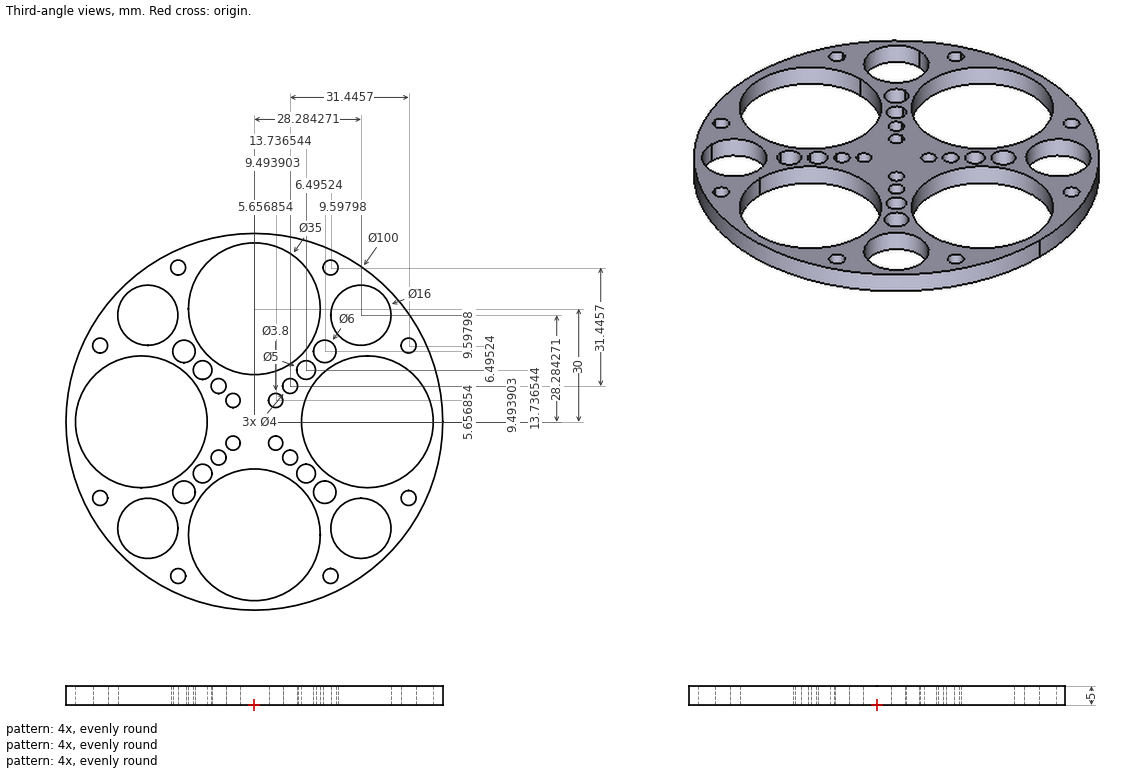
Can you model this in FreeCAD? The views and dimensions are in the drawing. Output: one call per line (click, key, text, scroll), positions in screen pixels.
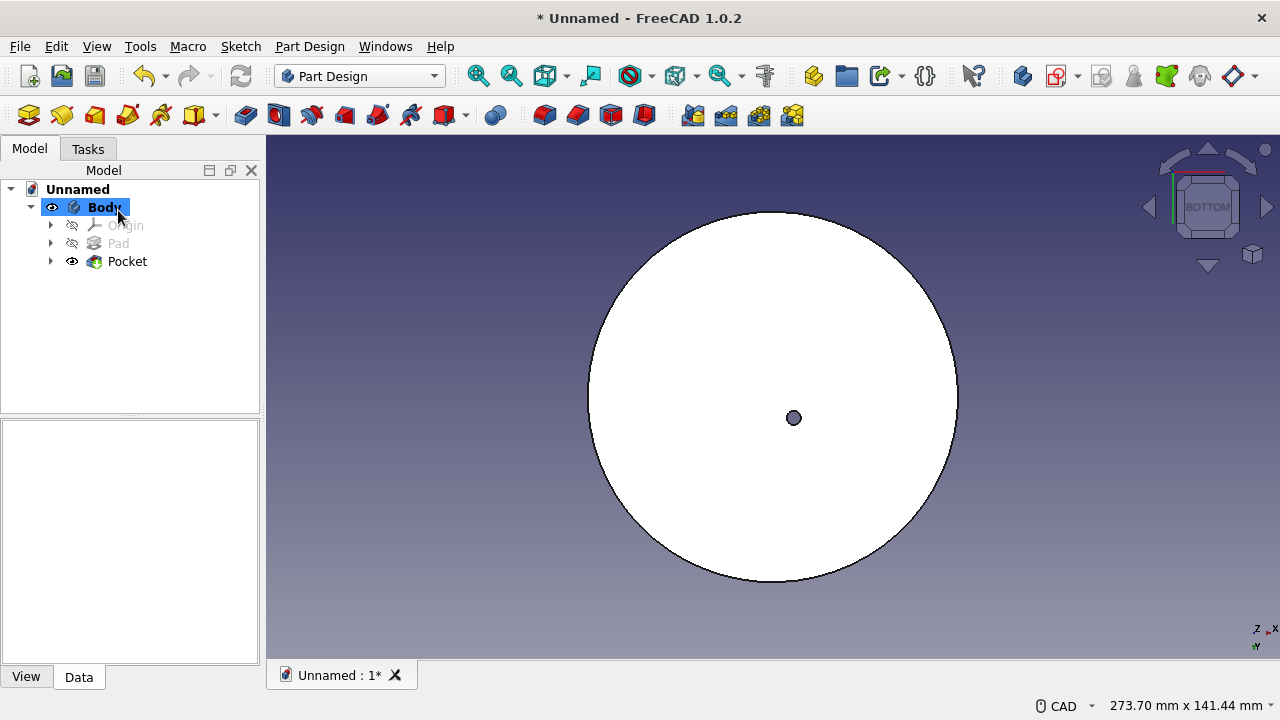
click(117, 261)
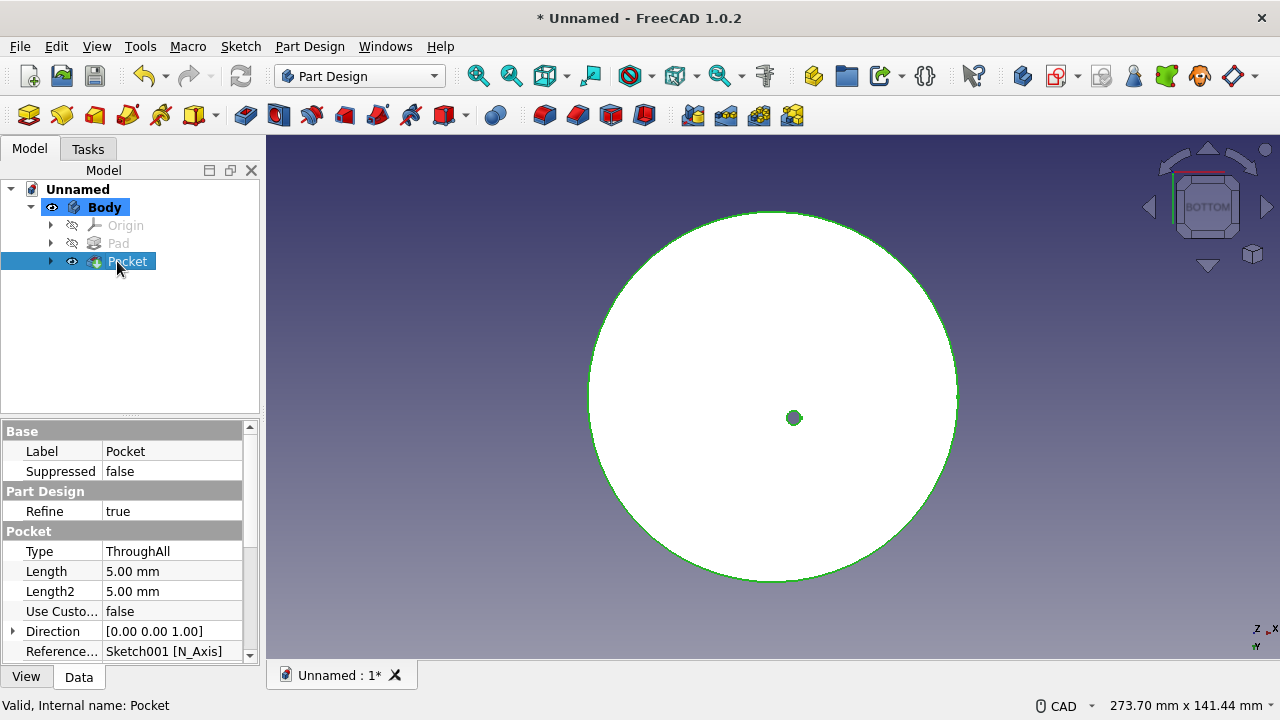
click(759, 116)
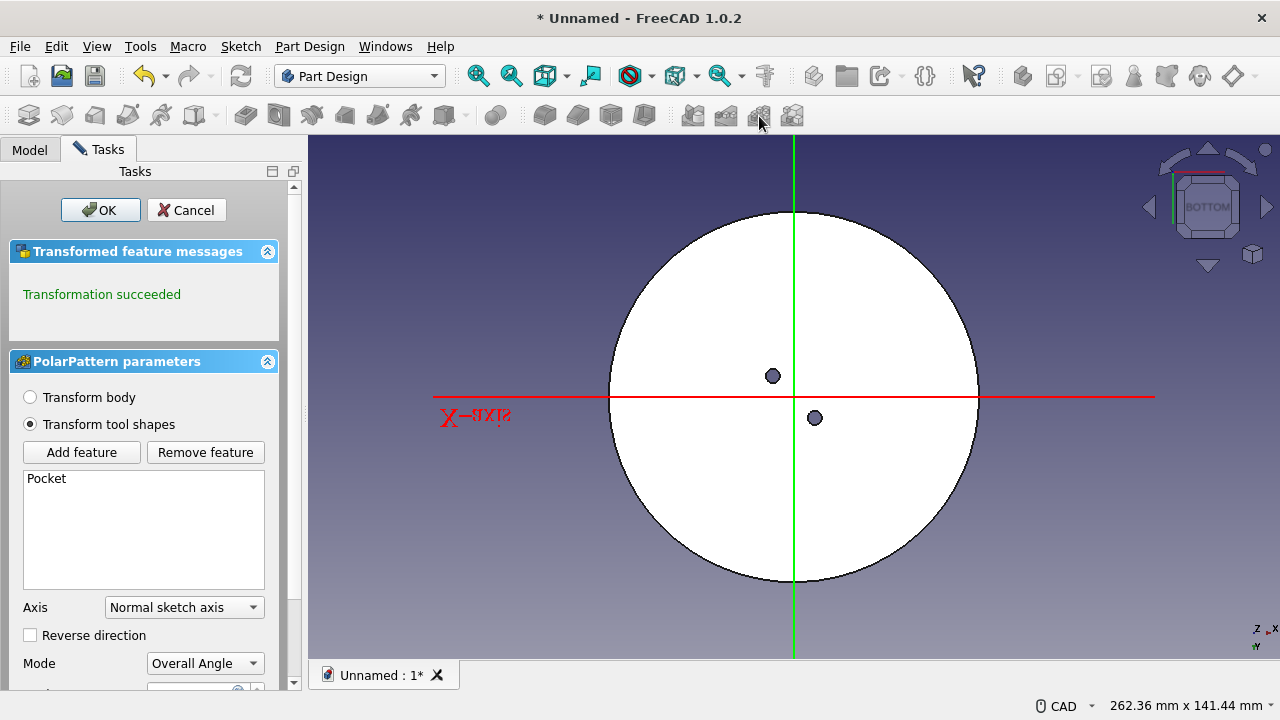
click(185, 608)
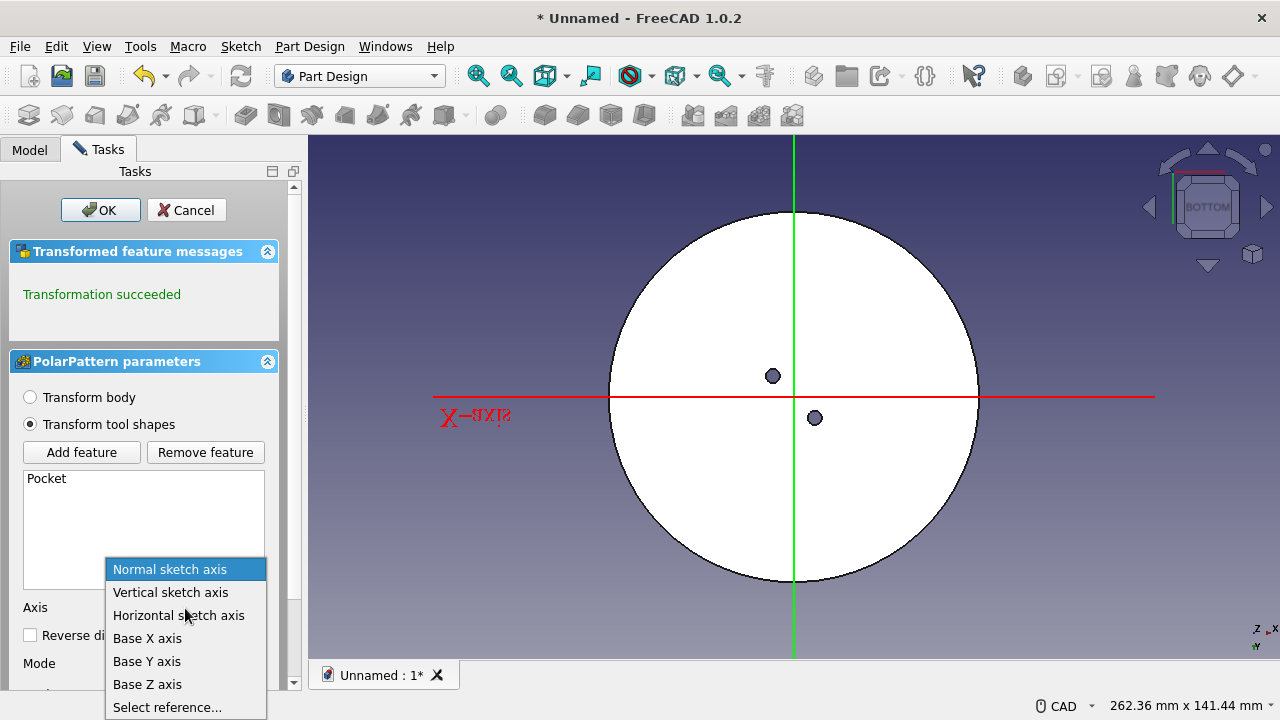
click(184, 684)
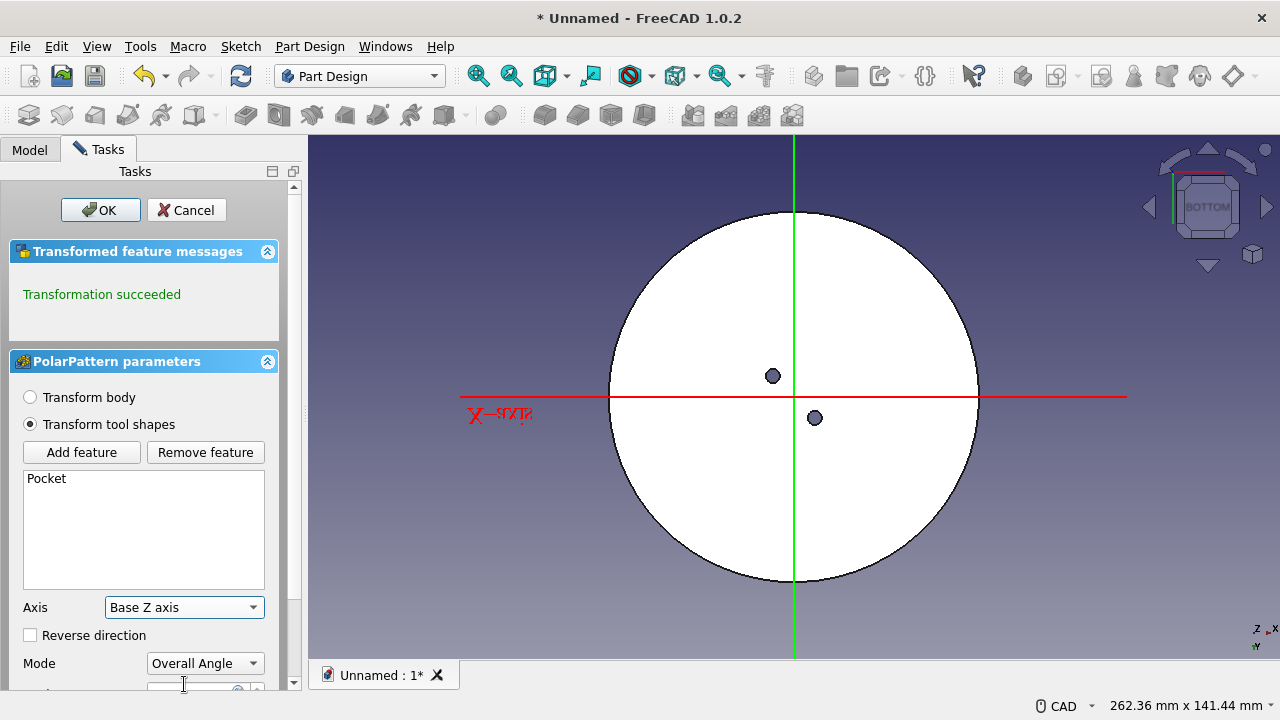
scroll(294, 436, down, 2)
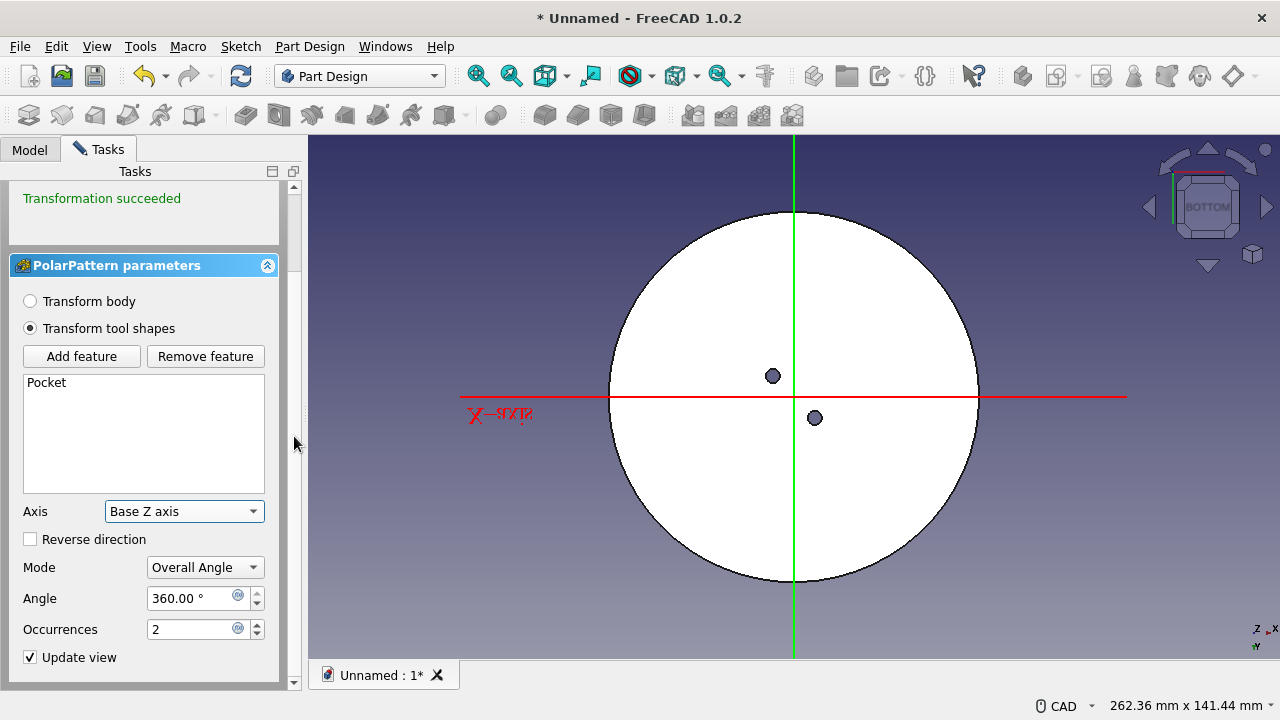
triple_click(199, 630)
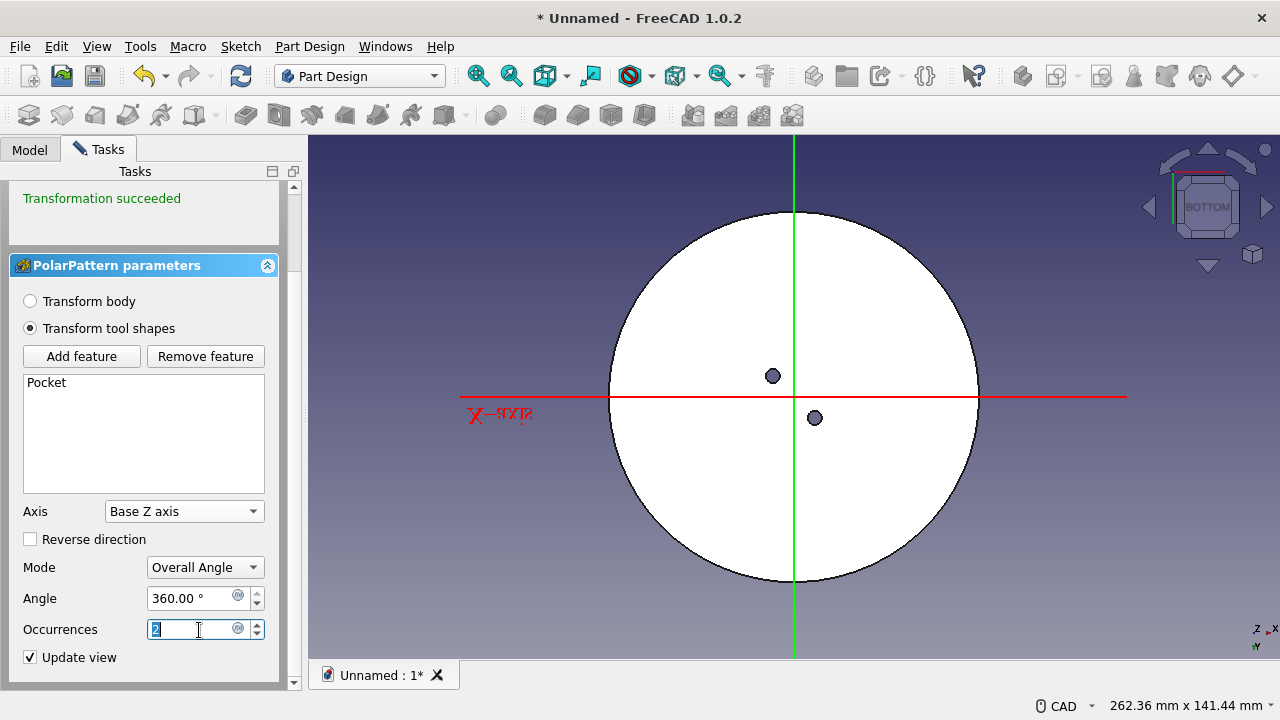
text(4)
key(Tab)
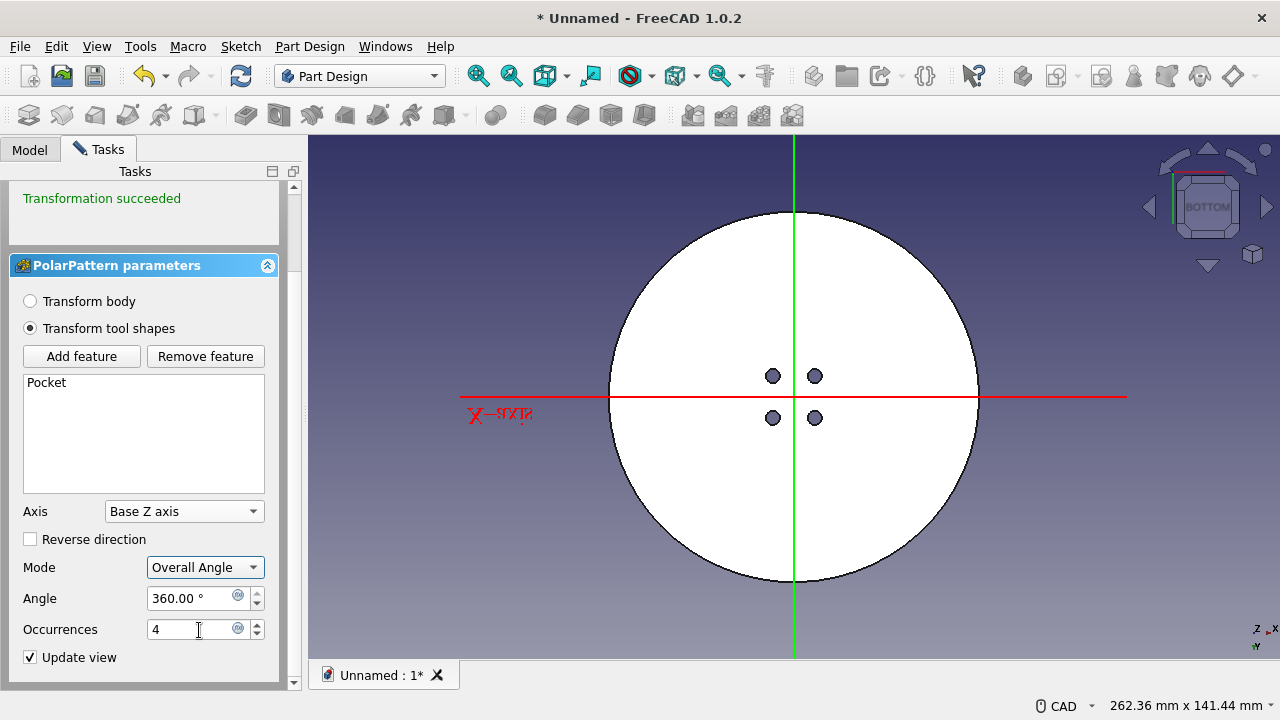
scroll(294, 436, up, 3)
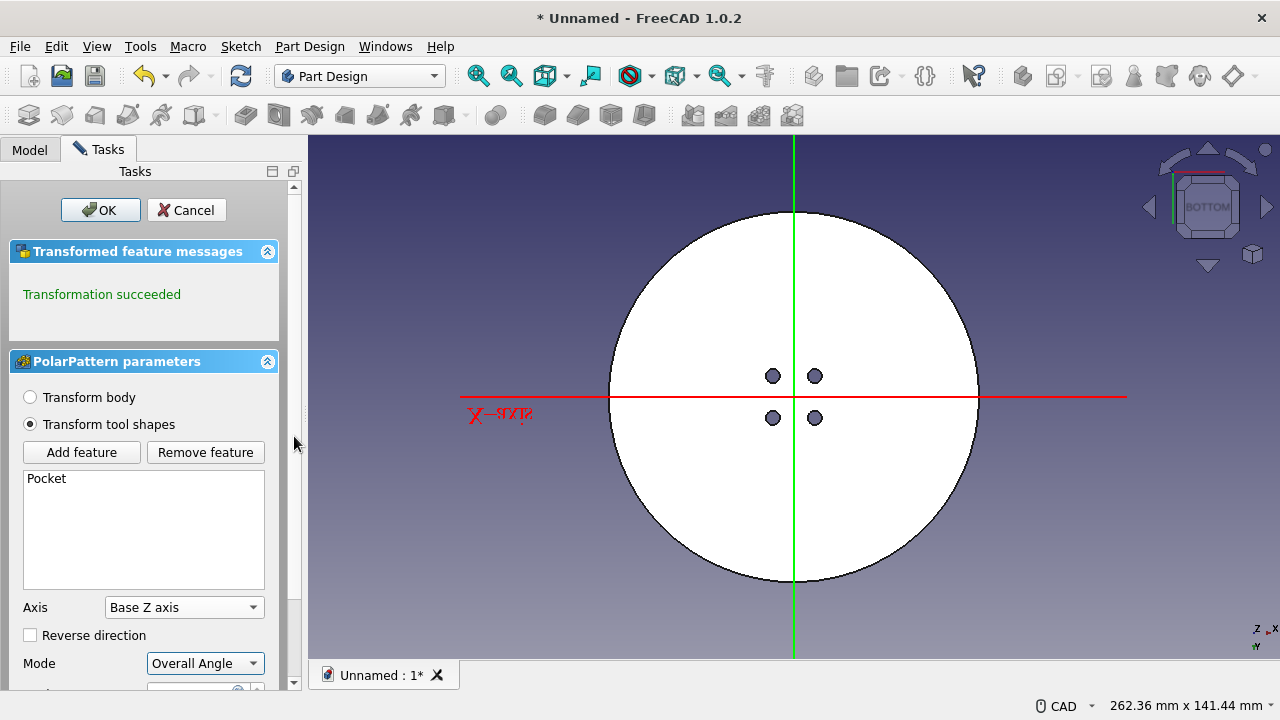
click(101, 210)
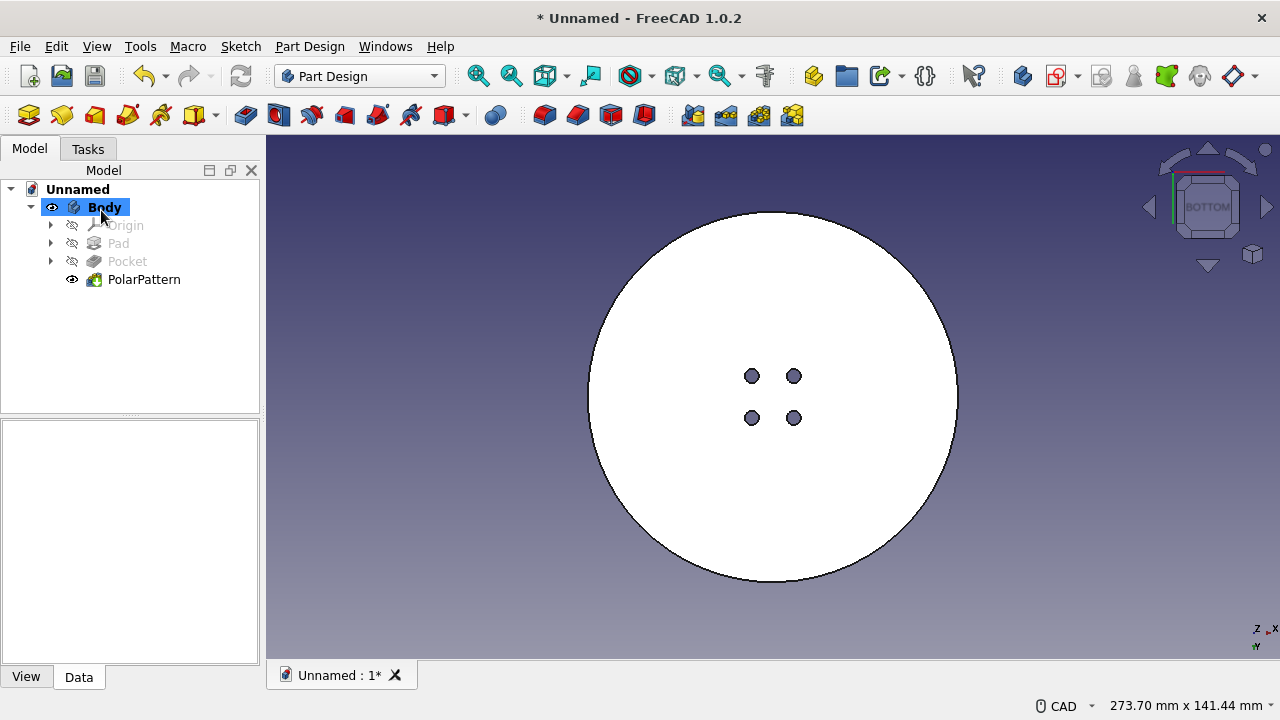
click(1056, 76)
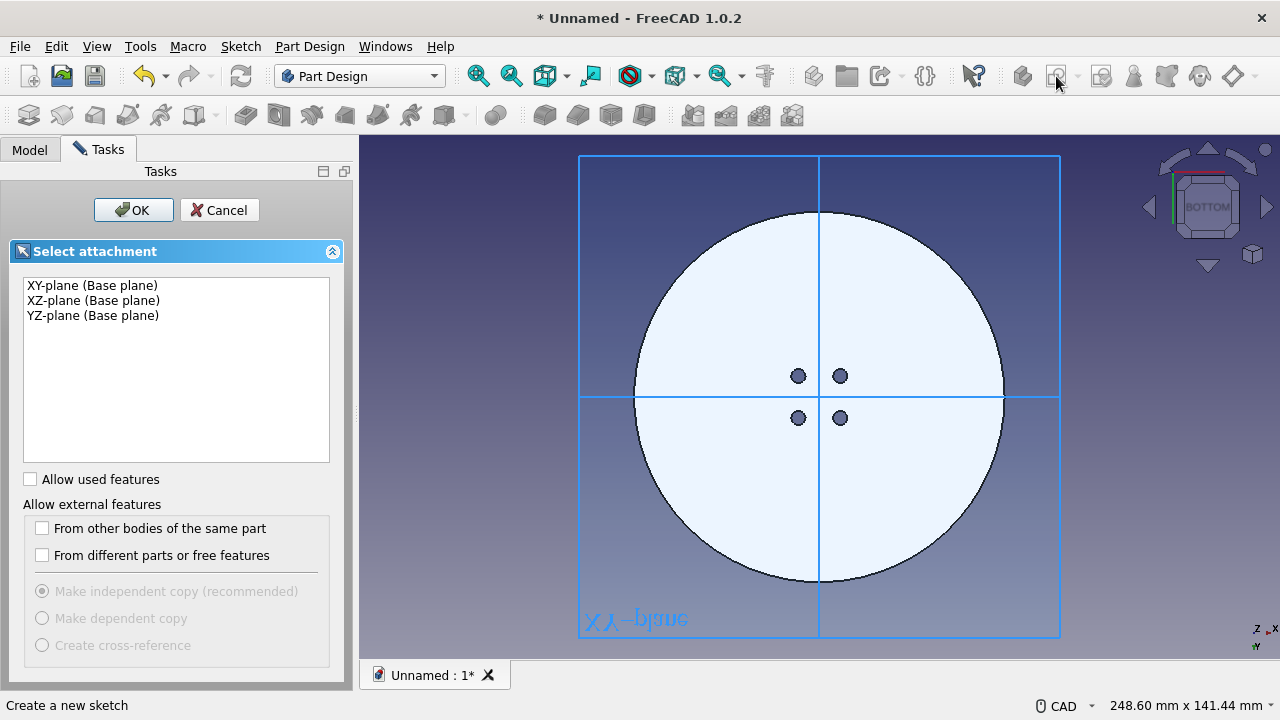
click(84, 286)